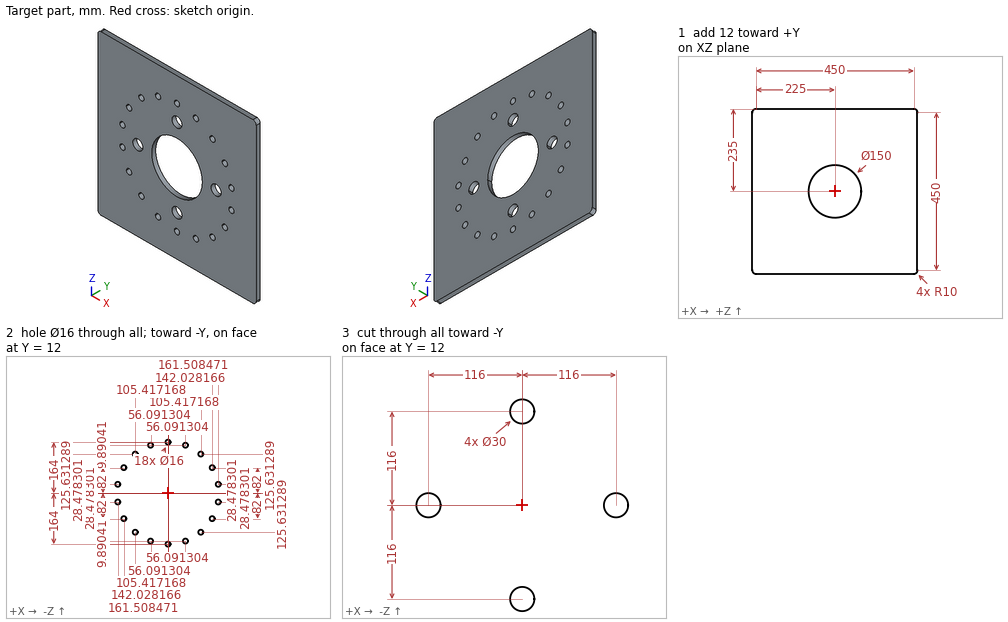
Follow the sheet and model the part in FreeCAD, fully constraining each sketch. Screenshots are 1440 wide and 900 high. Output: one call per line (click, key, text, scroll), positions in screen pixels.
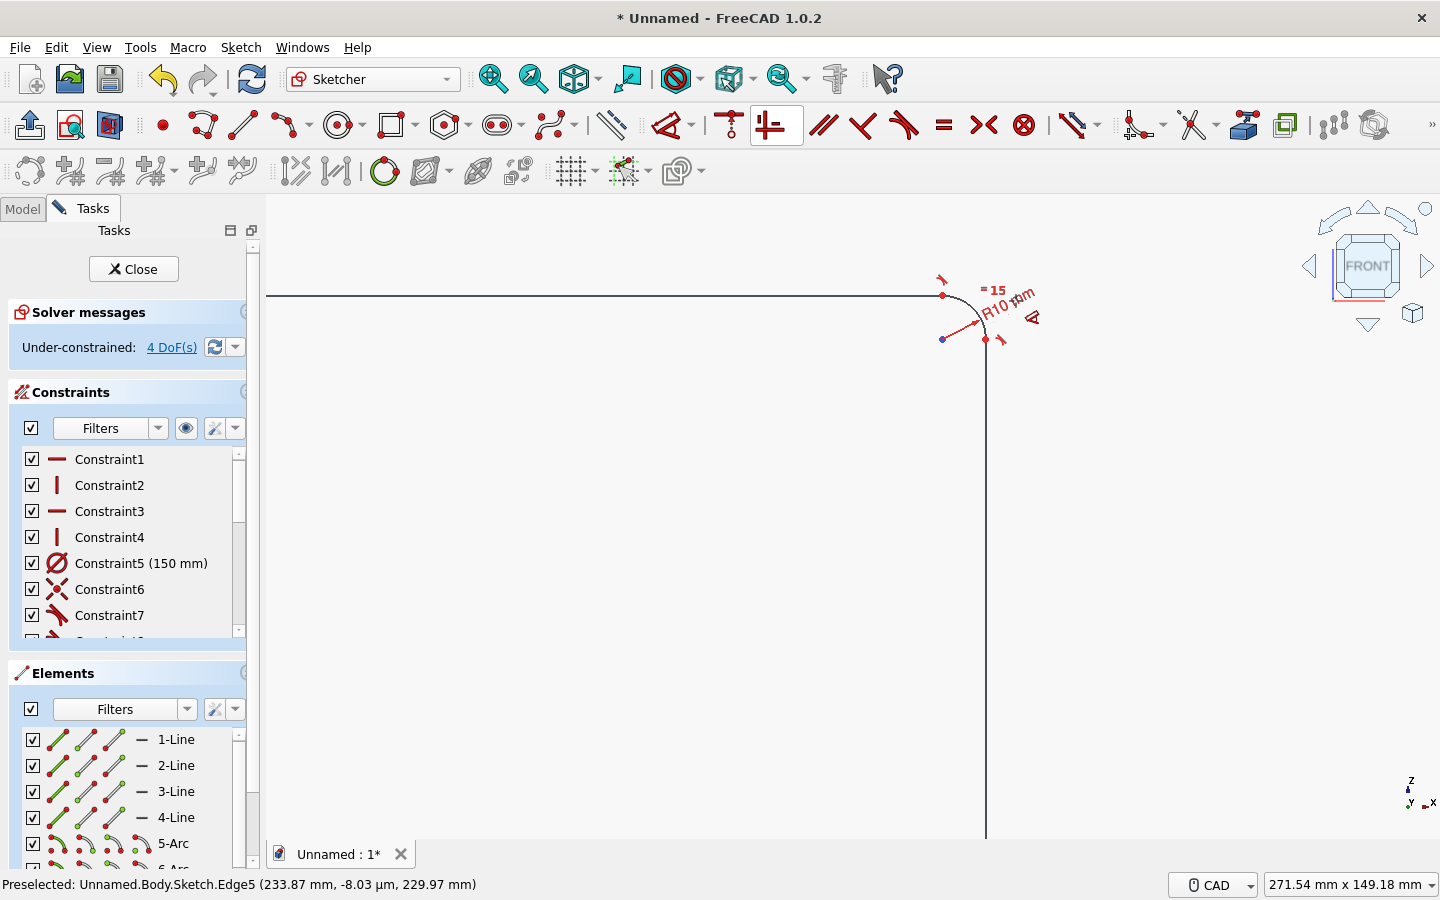
scroll(989, 316, down, 8)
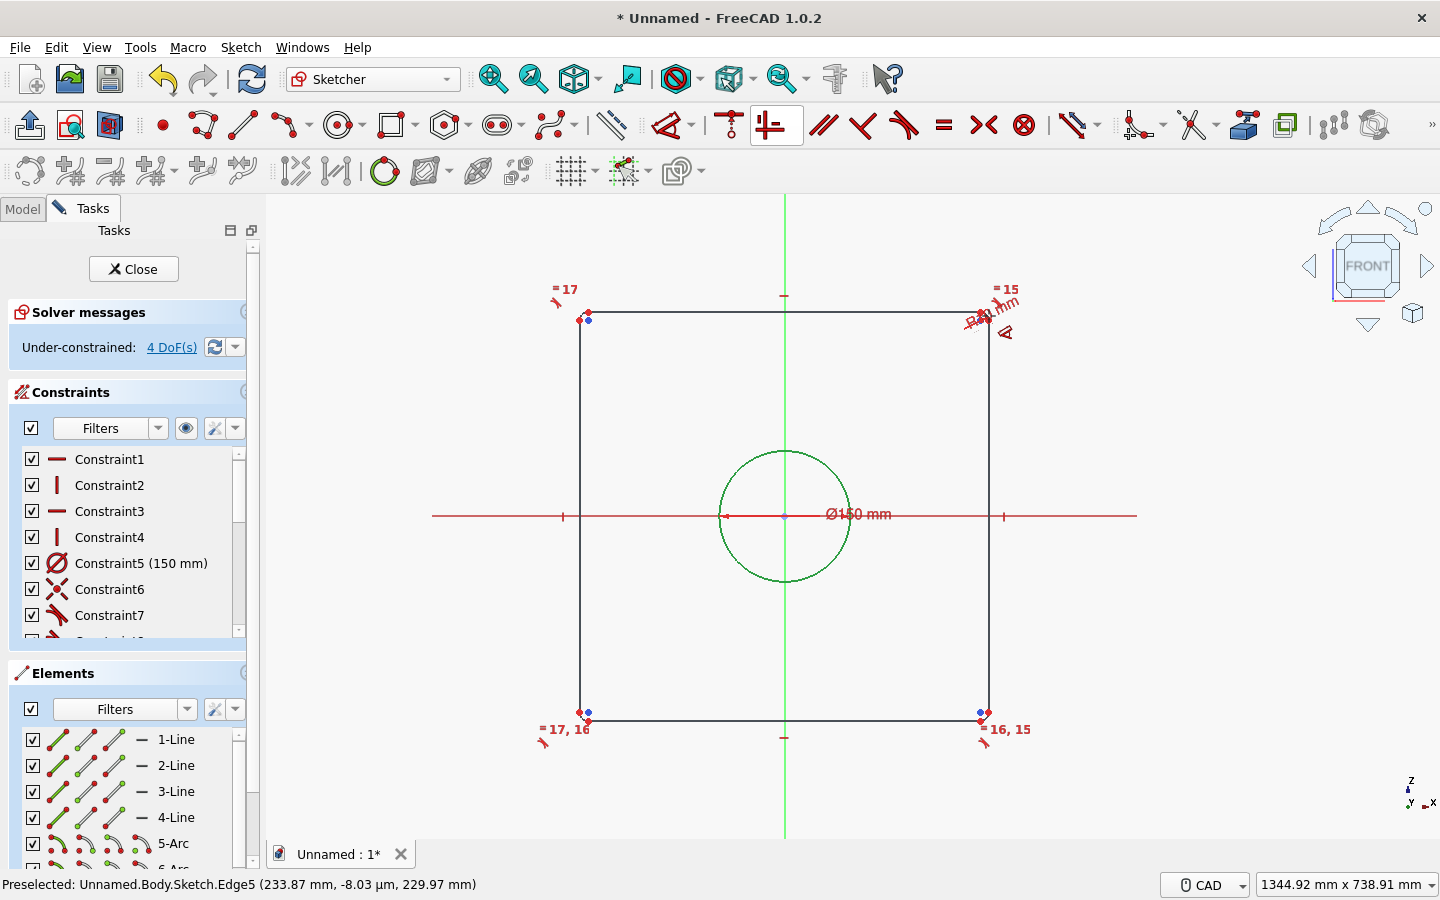
click(863, 312)
click(694, 278)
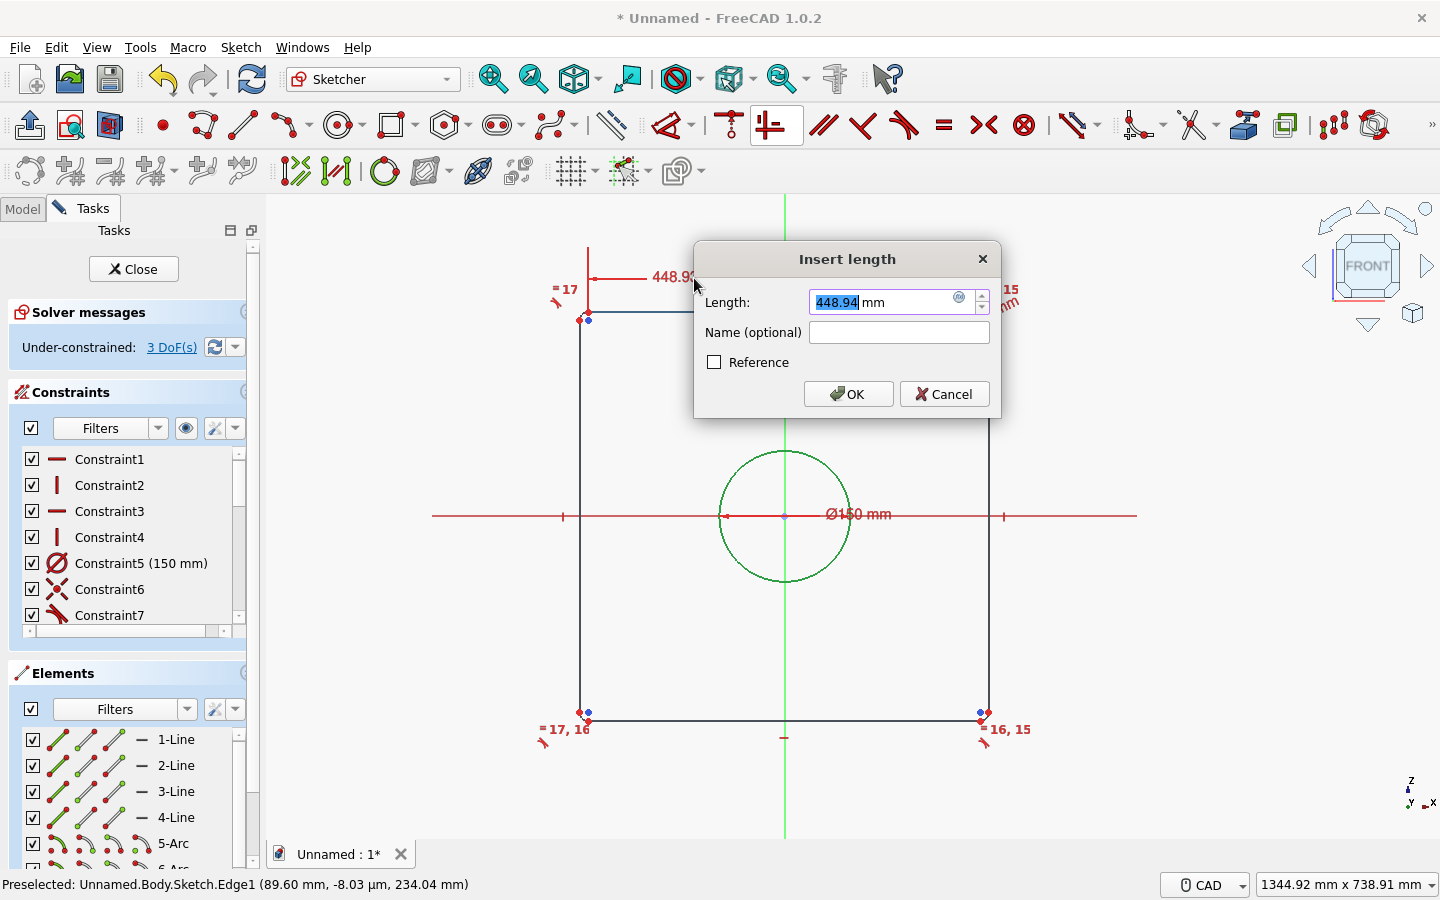
text(450)
key(Return)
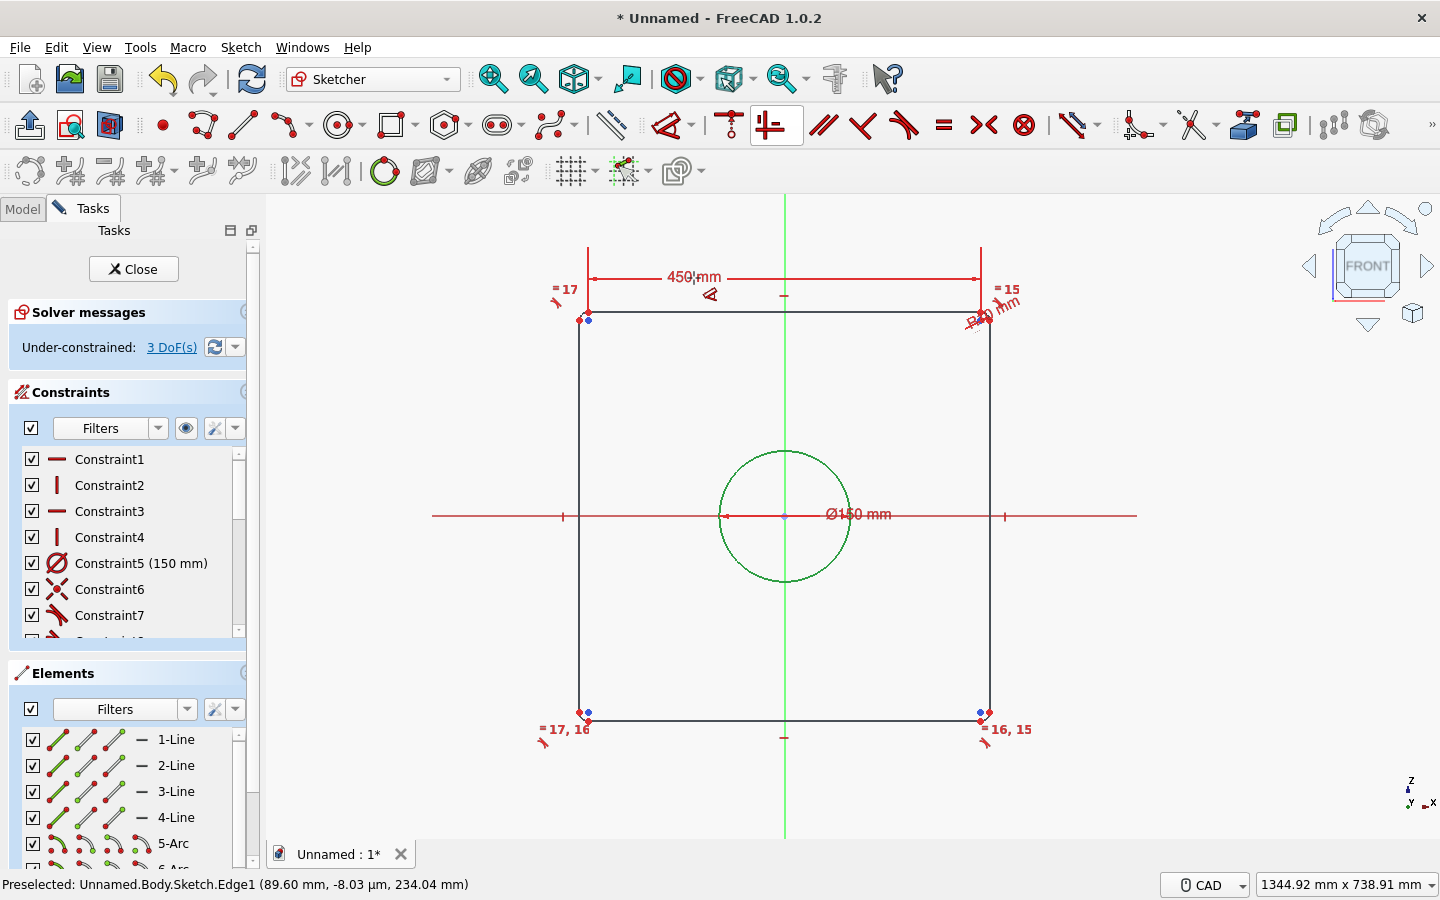
click(990, 438)
click(1024, 427)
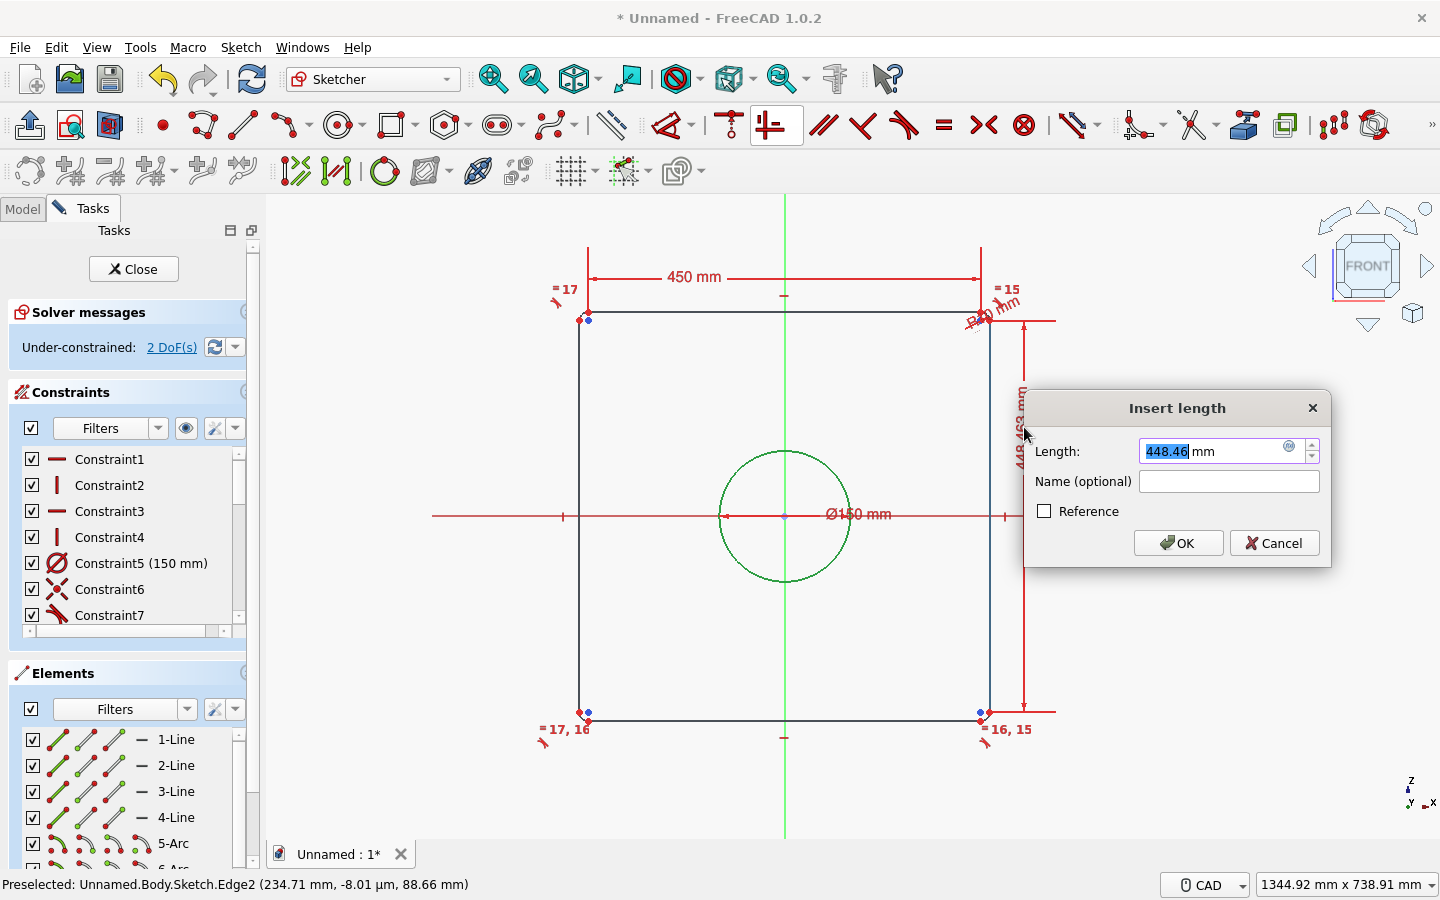
text(450)
key(Return)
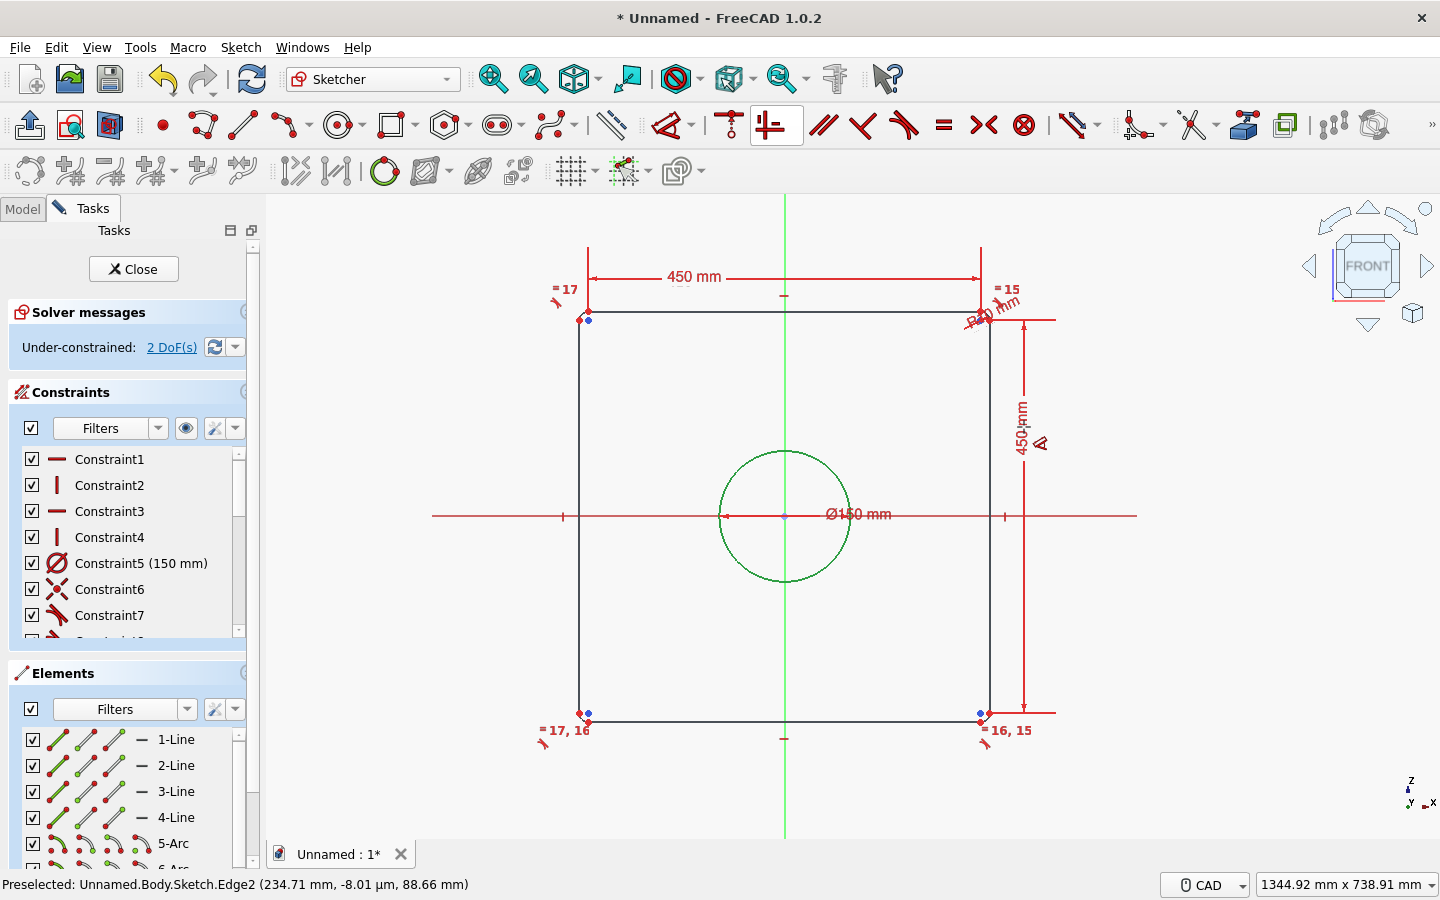
scroll(588, 312, up, 2)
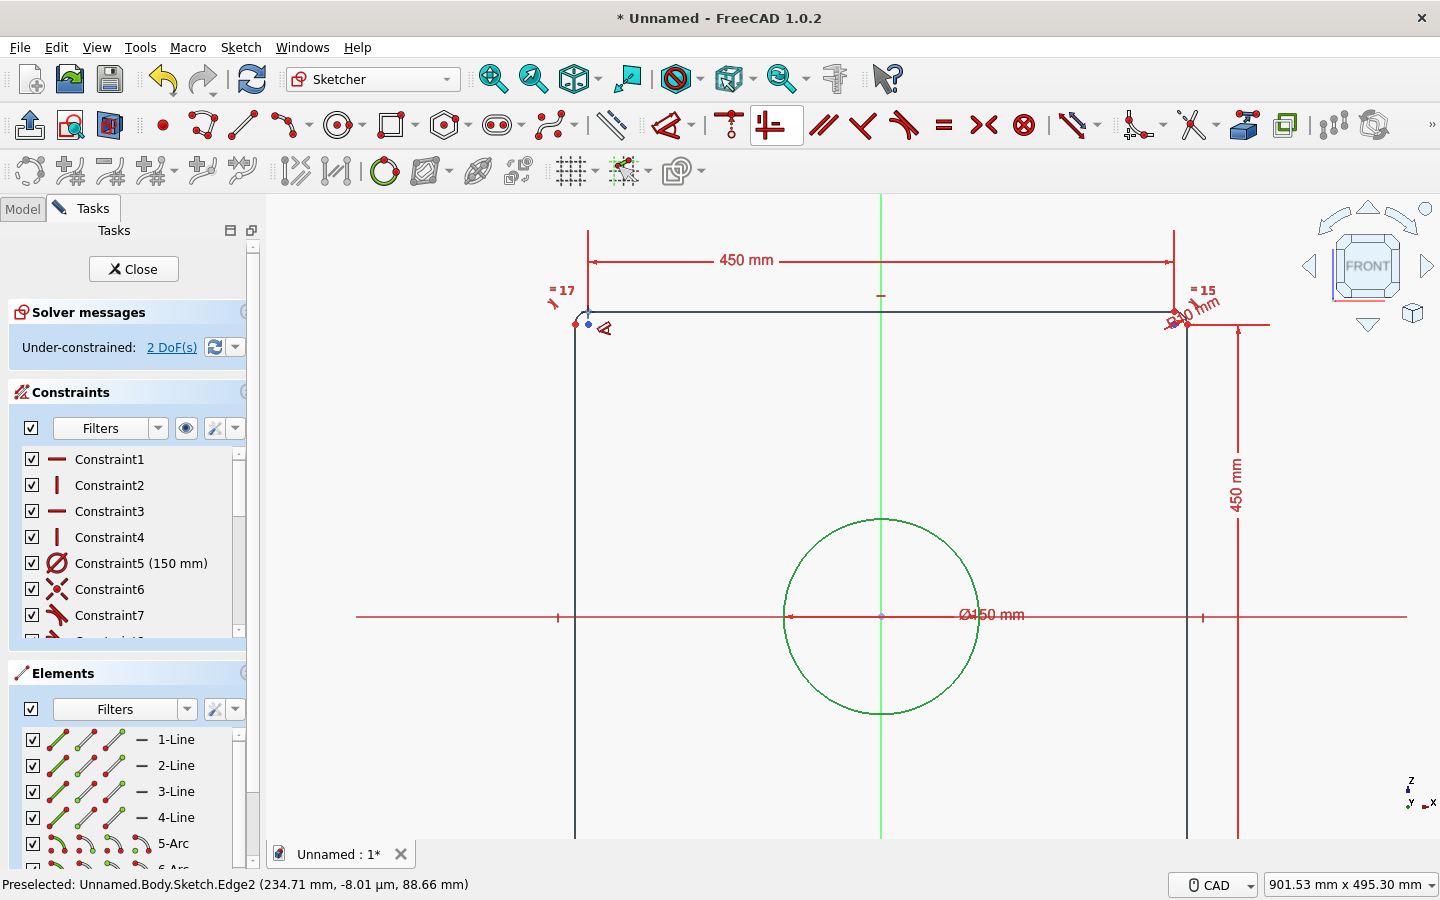
click(588, 312)
click(667, 278)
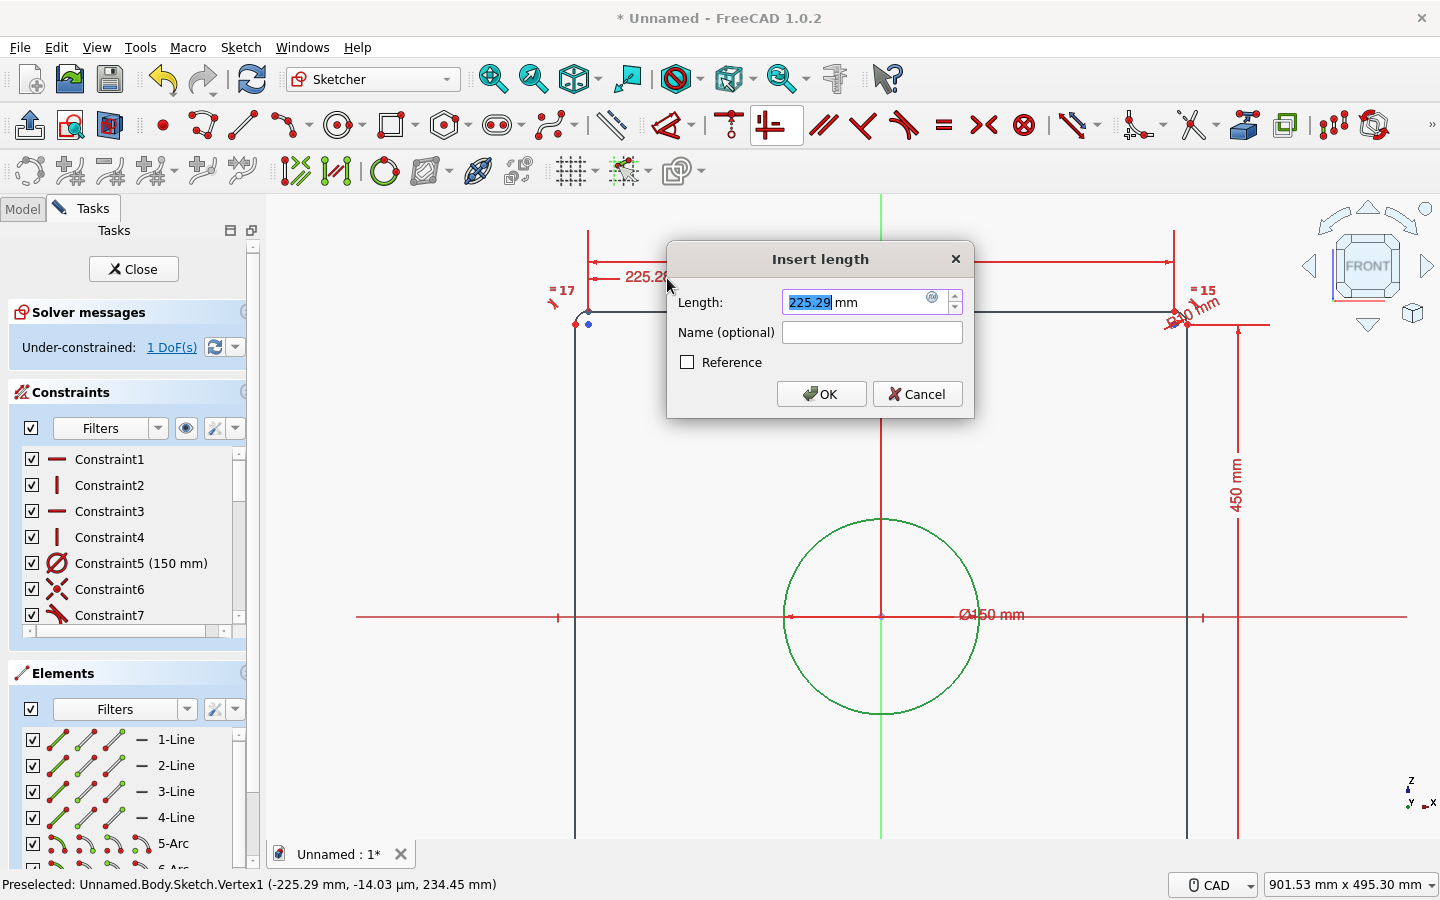
text(225)
key(Return)